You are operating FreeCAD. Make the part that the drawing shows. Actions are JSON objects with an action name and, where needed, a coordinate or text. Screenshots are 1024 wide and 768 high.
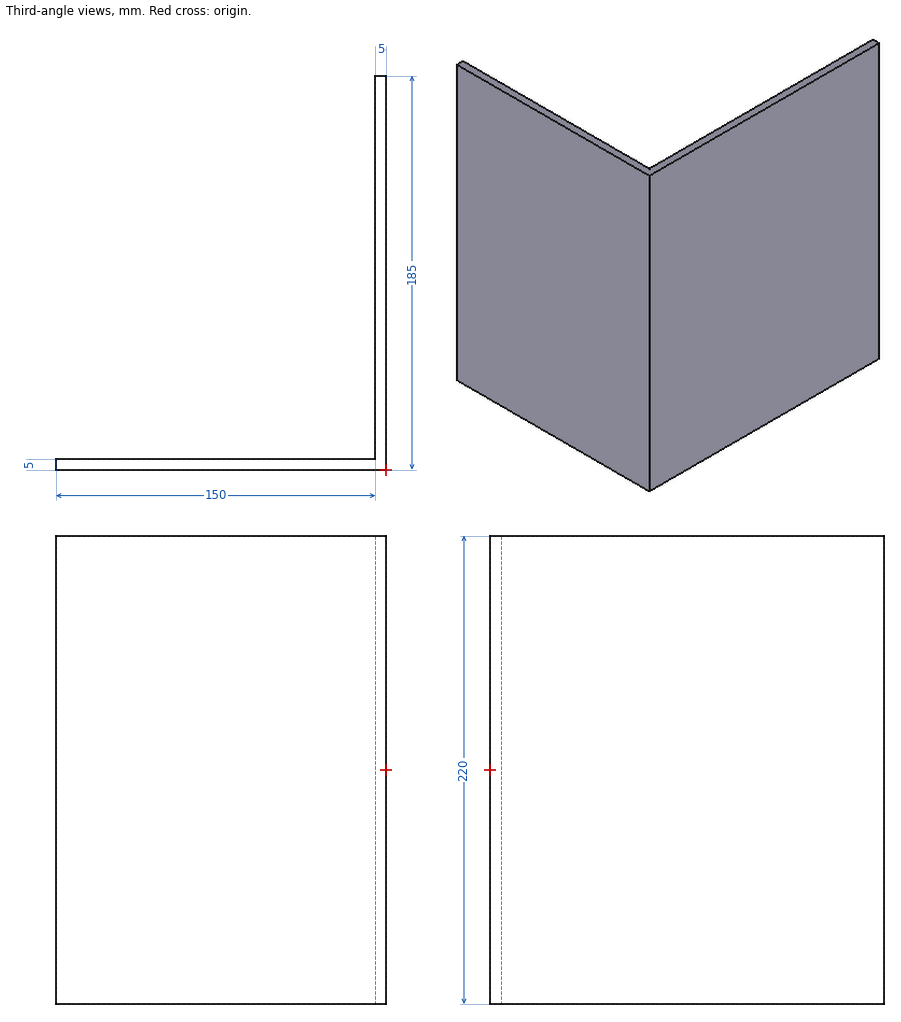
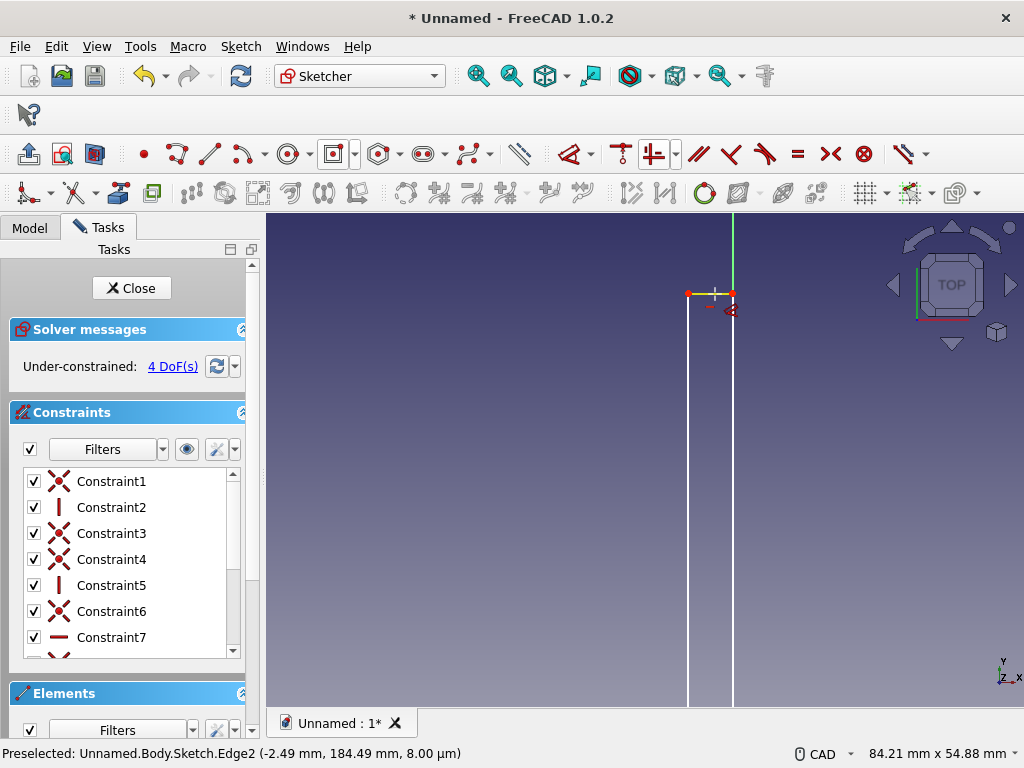
{"action": "left_click", "coordinate": [715, 294]}
{"action": "left_click", "coordinate": [710, 260]}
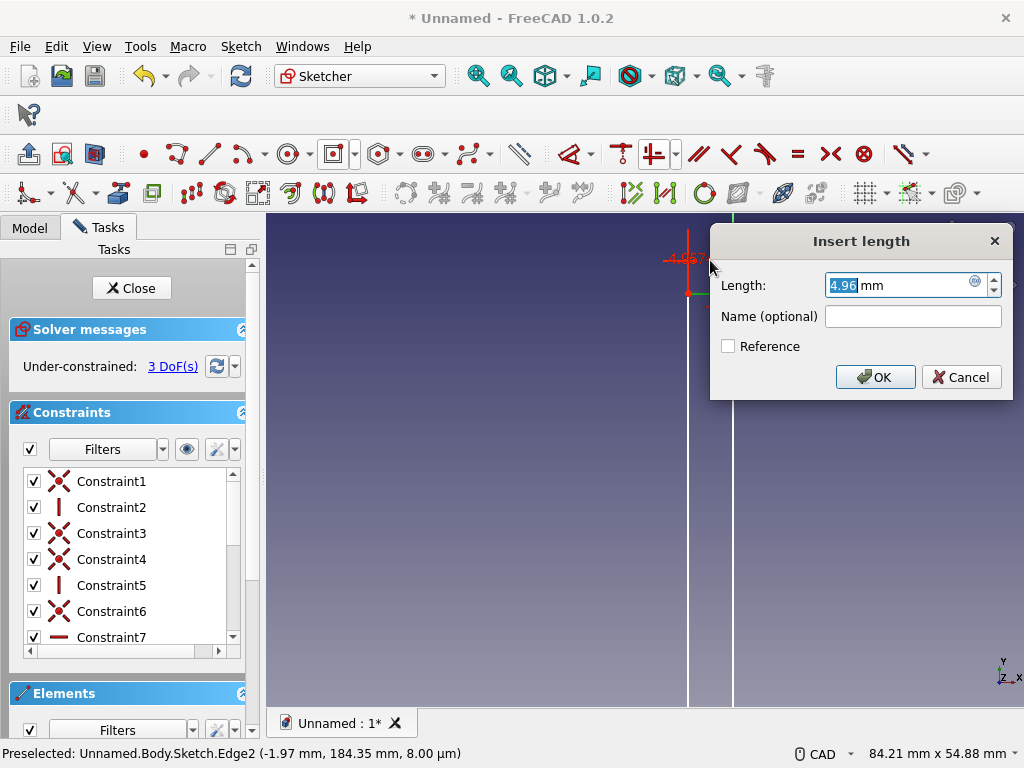
{"action": "type", "text": "5"}
{"action": "key", "text": "Return"}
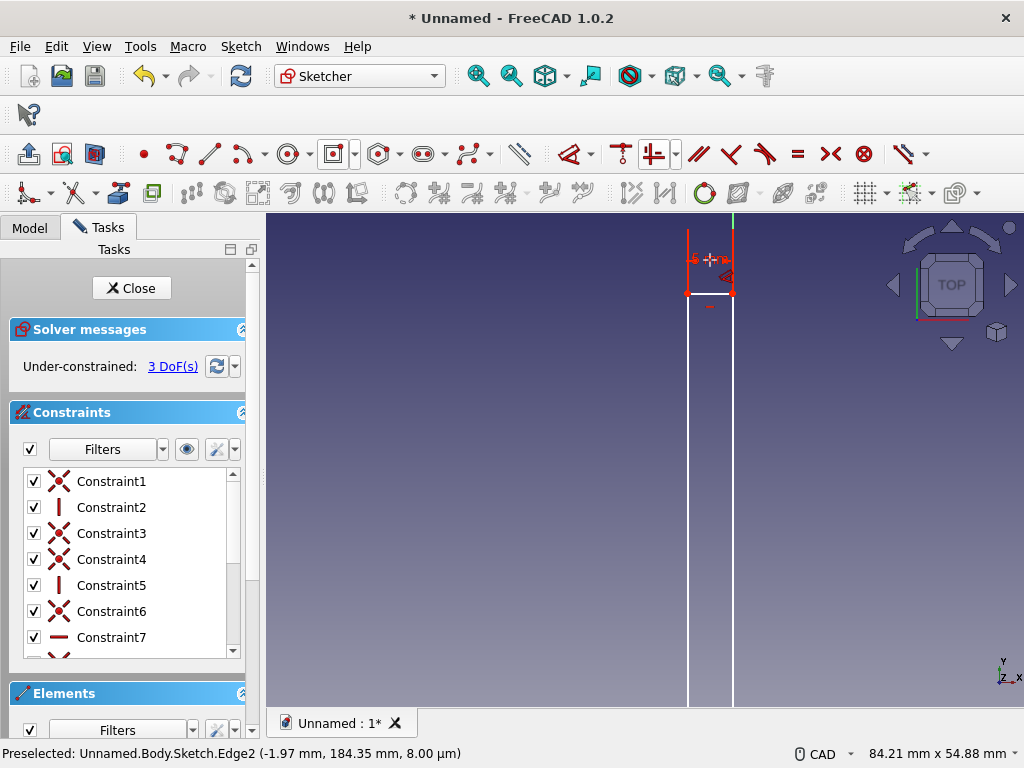
{"action": "scroll", "coordinate": [713, 293], "scroll_direction": "down", "scroll_amount": 8}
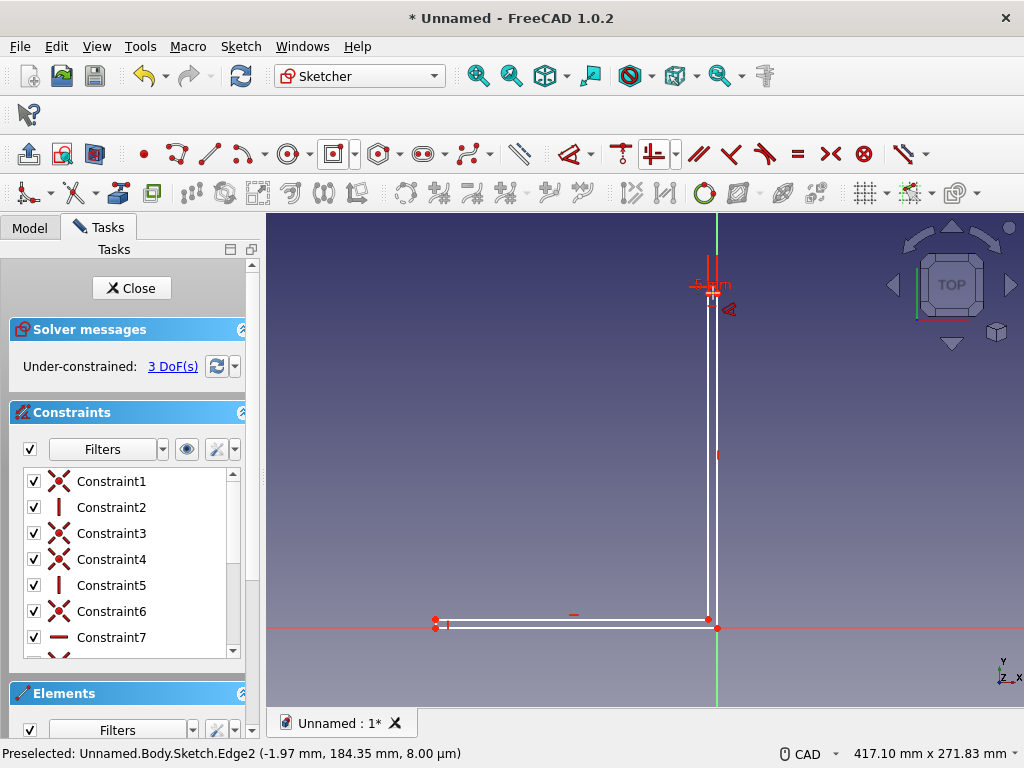
{"action": "scroll", "coordinate": [436, 622], "scroll_direction": "up", "scroll_amount": 9}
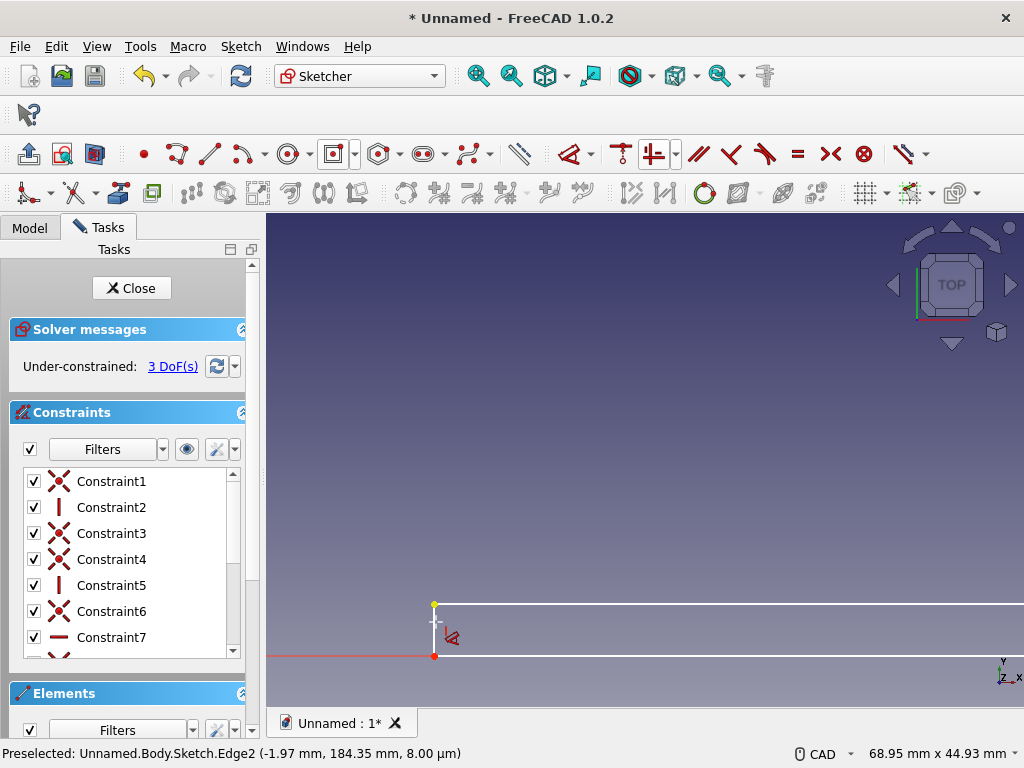
{"action": "left_click", "coordinate": [434, 620]}
{"action": "left_click", "coordinate": [400, 630]}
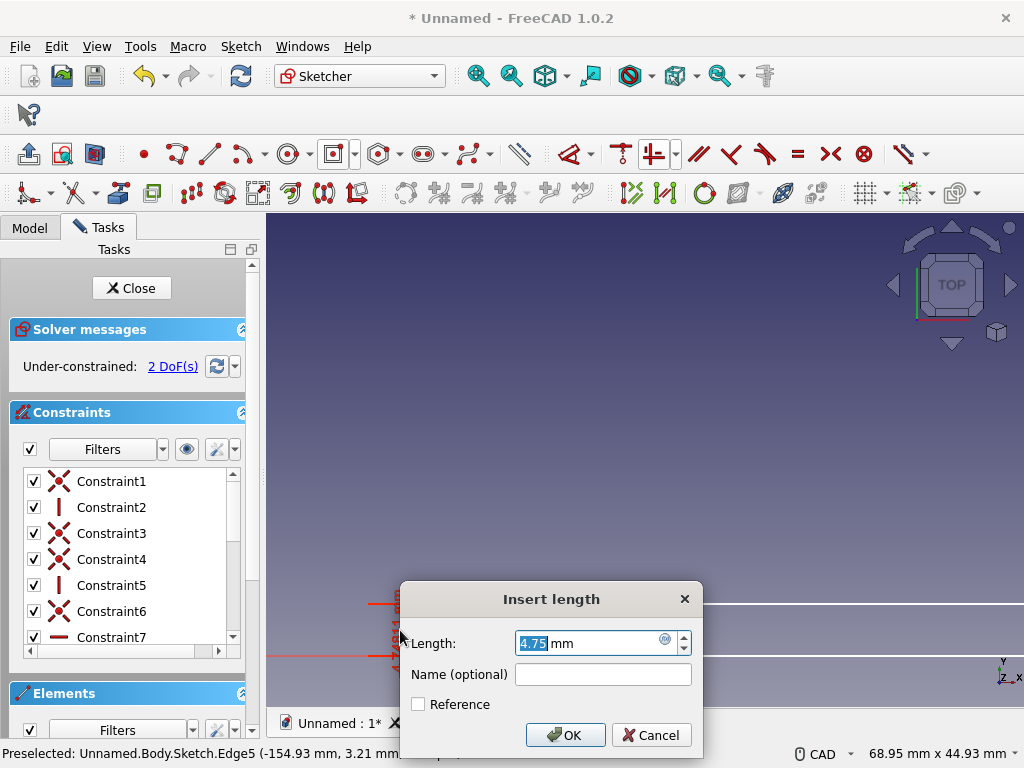
{"action": "type", "text": "5"}
{"action": "key", "text": "Return"}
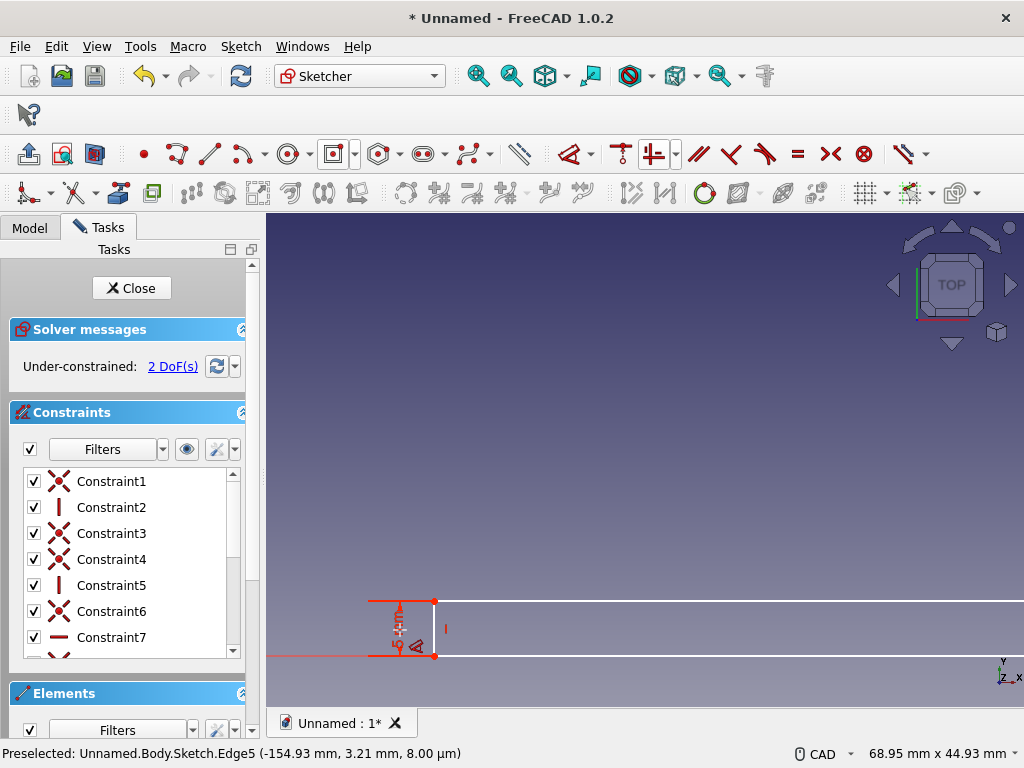
{"action": "scroll", "coordinate": [436, 623], "scroll_direction": "down", "scroll_amount": 9}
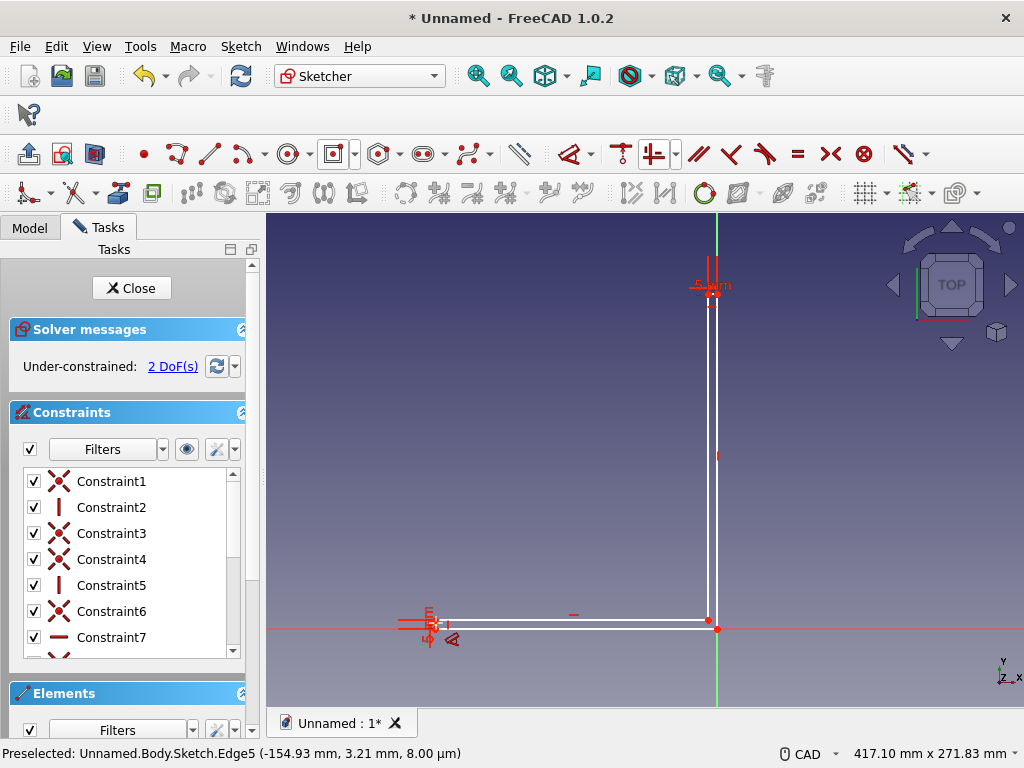
{"action": "scroll", "coordinate": [717, 529], "scroll_direction": "up", "scroll_amount": 3}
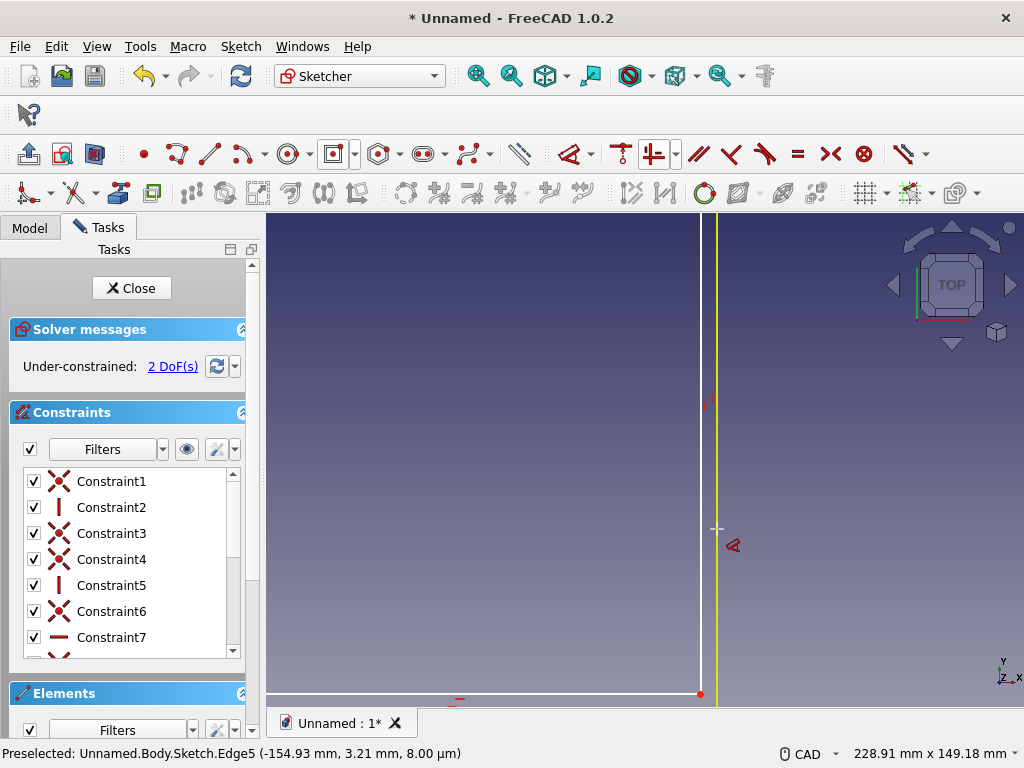
{"action": "left_click", "coordinate": [717, 528]}
{"action": "left_click", "coordinate": [751, 460]}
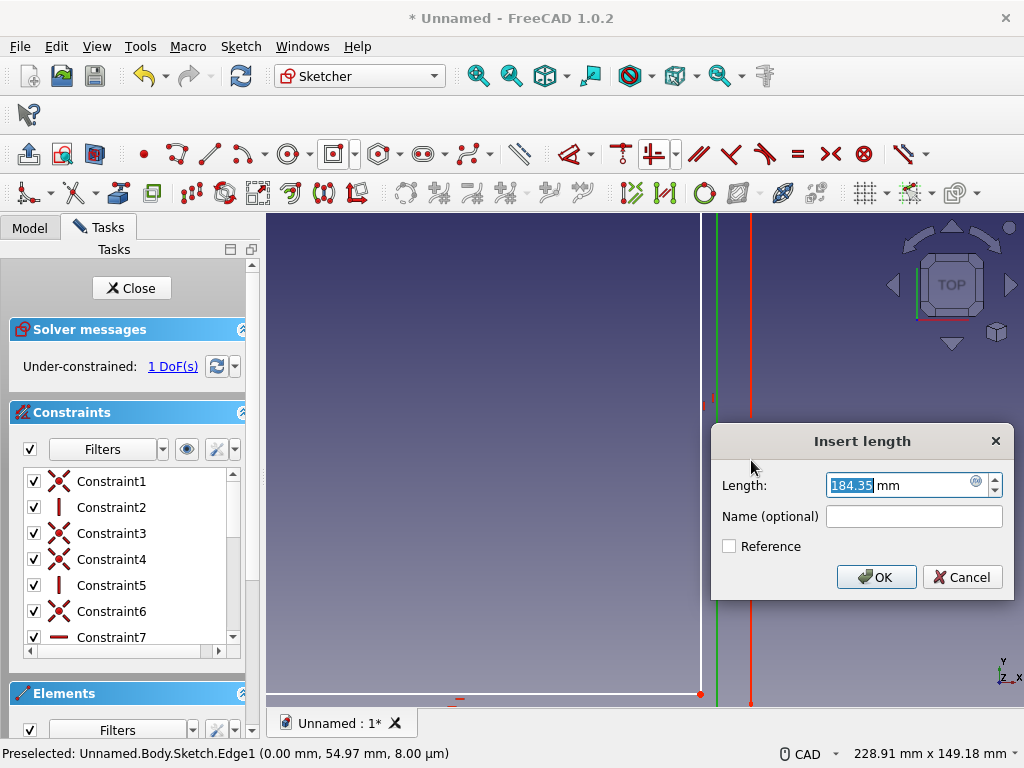
{"action": "type", "text": "185"}
{"action": "key", "text": "Return"}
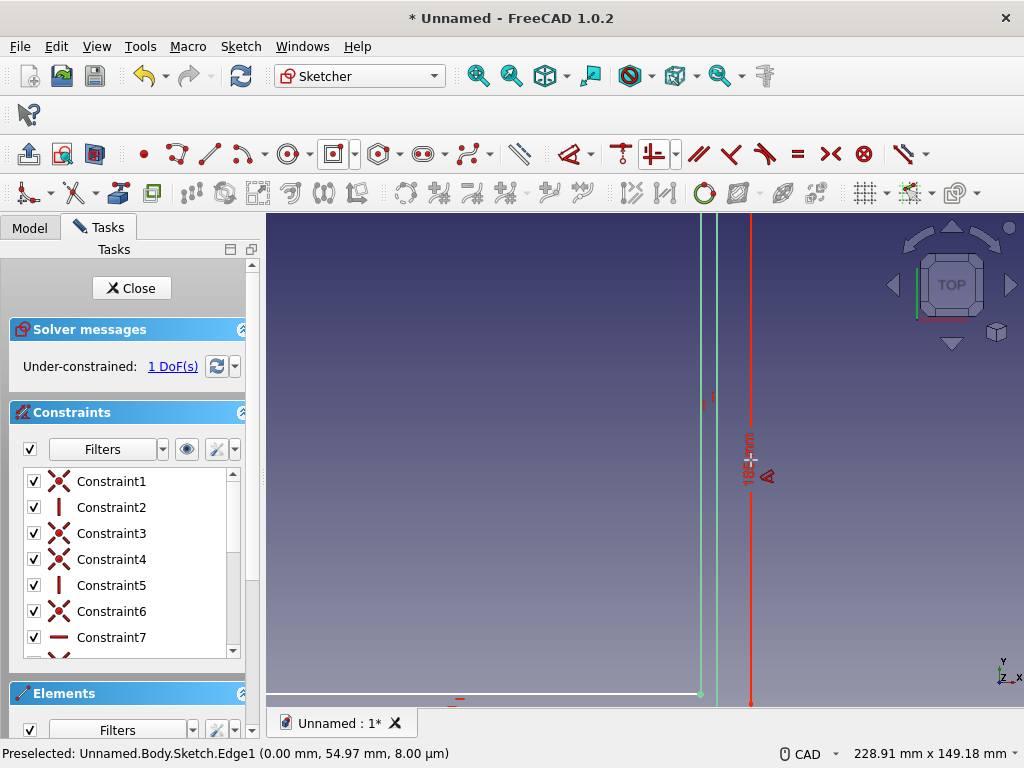
{"action": "scroll", "coordinate": [717, 527], "scroll_direction": "down", "scroll_amount": 3}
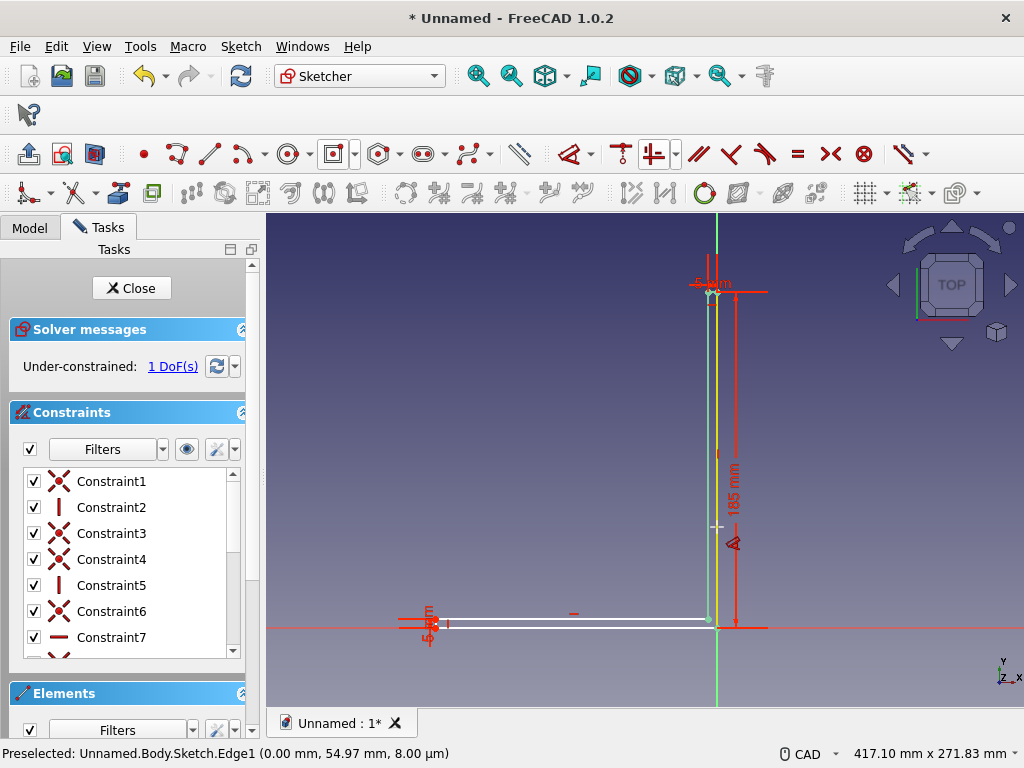
{"action": "scroll", "coordinate": [627, 619], "scroll_direction": "up", "scroll_amount": 3}